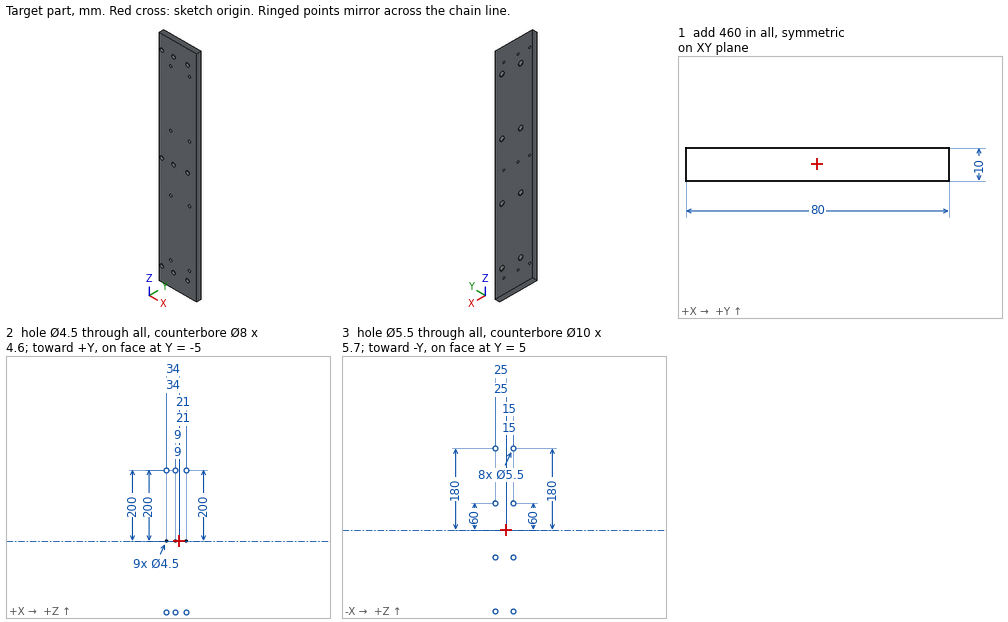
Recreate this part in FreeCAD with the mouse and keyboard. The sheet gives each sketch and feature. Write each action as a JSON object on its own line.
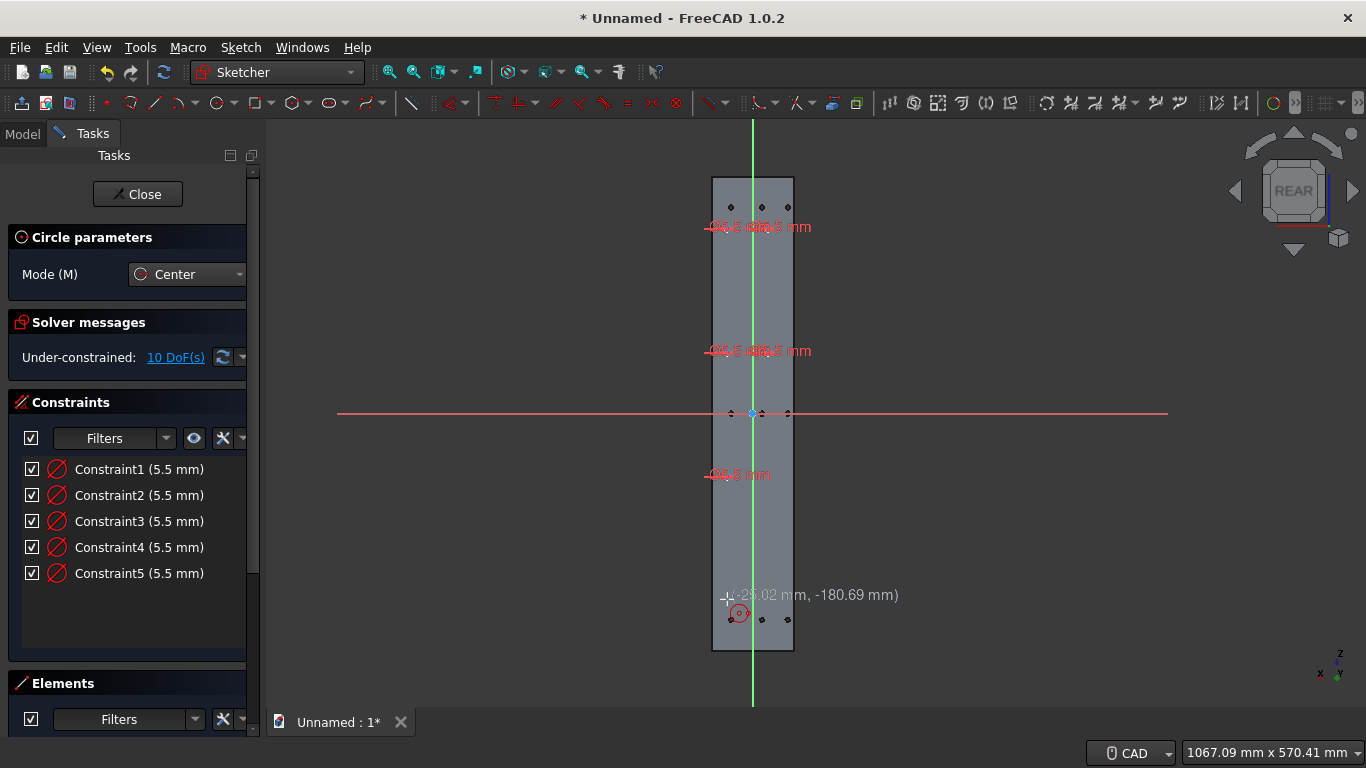
{"action": "left_click", "coordinate": [727, 599]}
{"action": "mouse_move", "coordinate": [729, 597]}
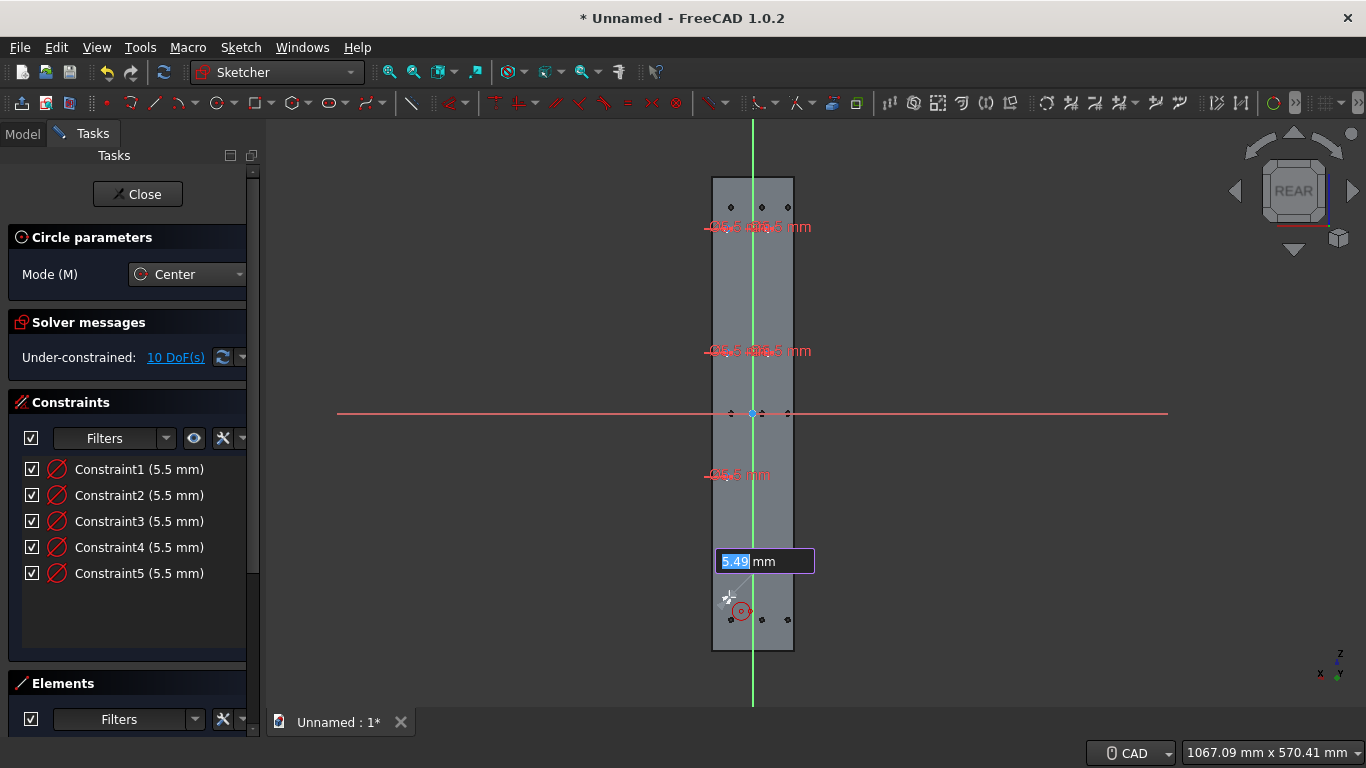
{"action": "type", "text": "5.5"}
{"action": "key", "text": "Return"}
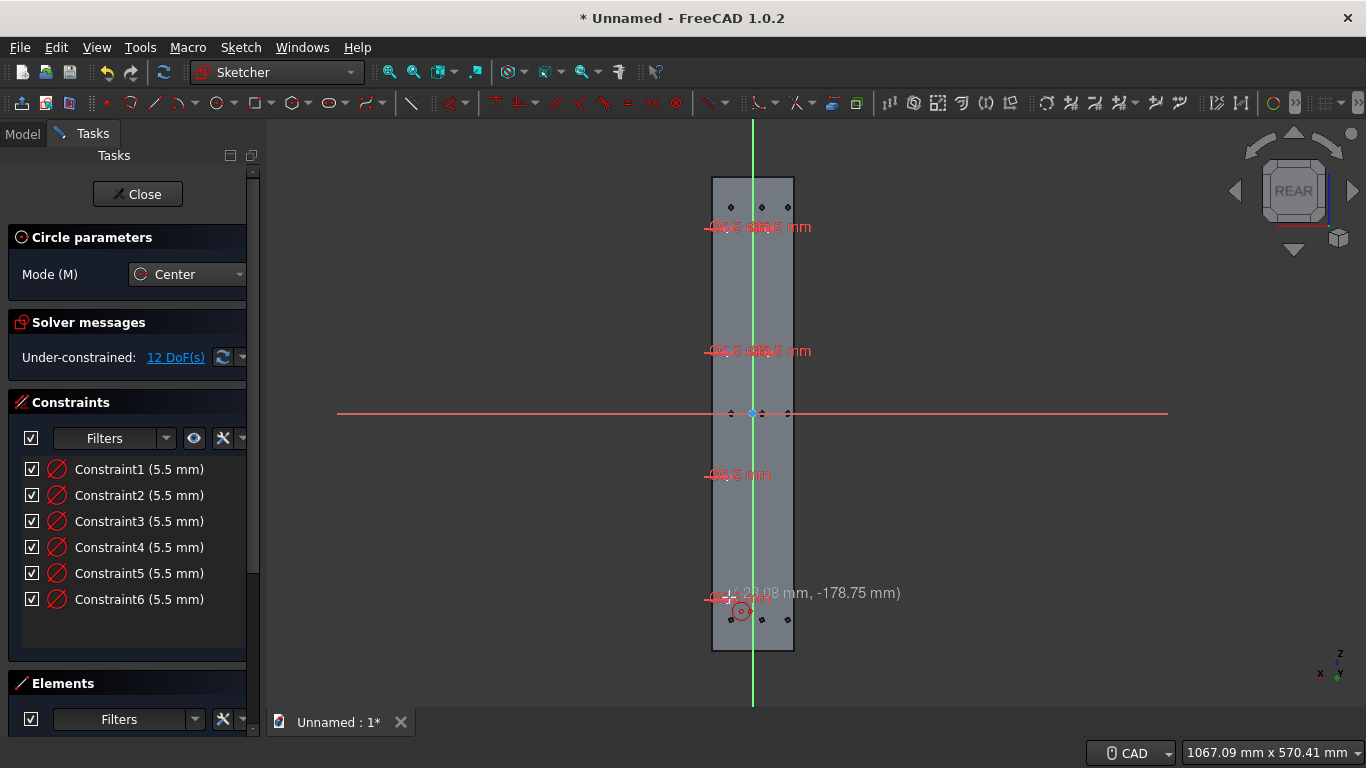
{"action": "scroll", "coordinate": [768, 599], "scroll_direction": "up", "scroll_amount": 11}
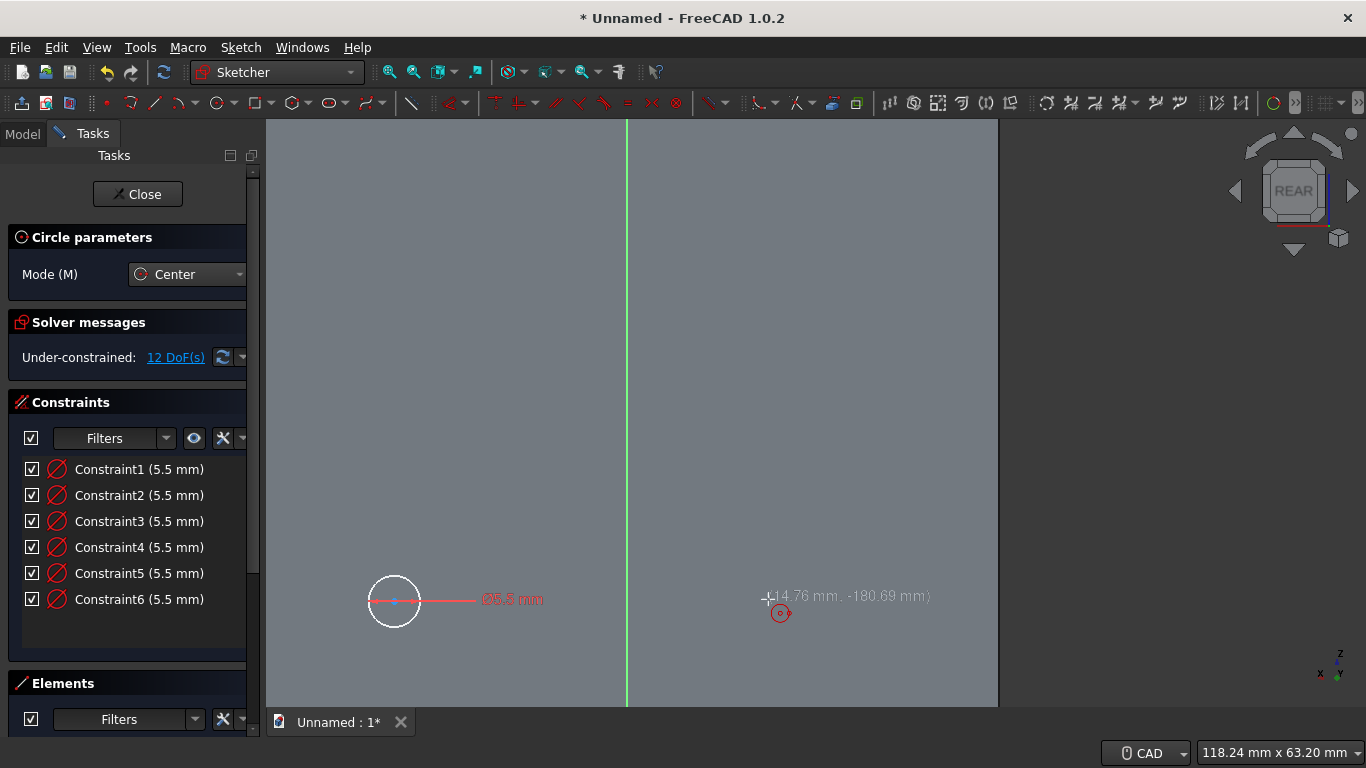
{"action": "scroll", "coordinate": [768, 599], "scroll_direction": "down", "scroll_amount": 11}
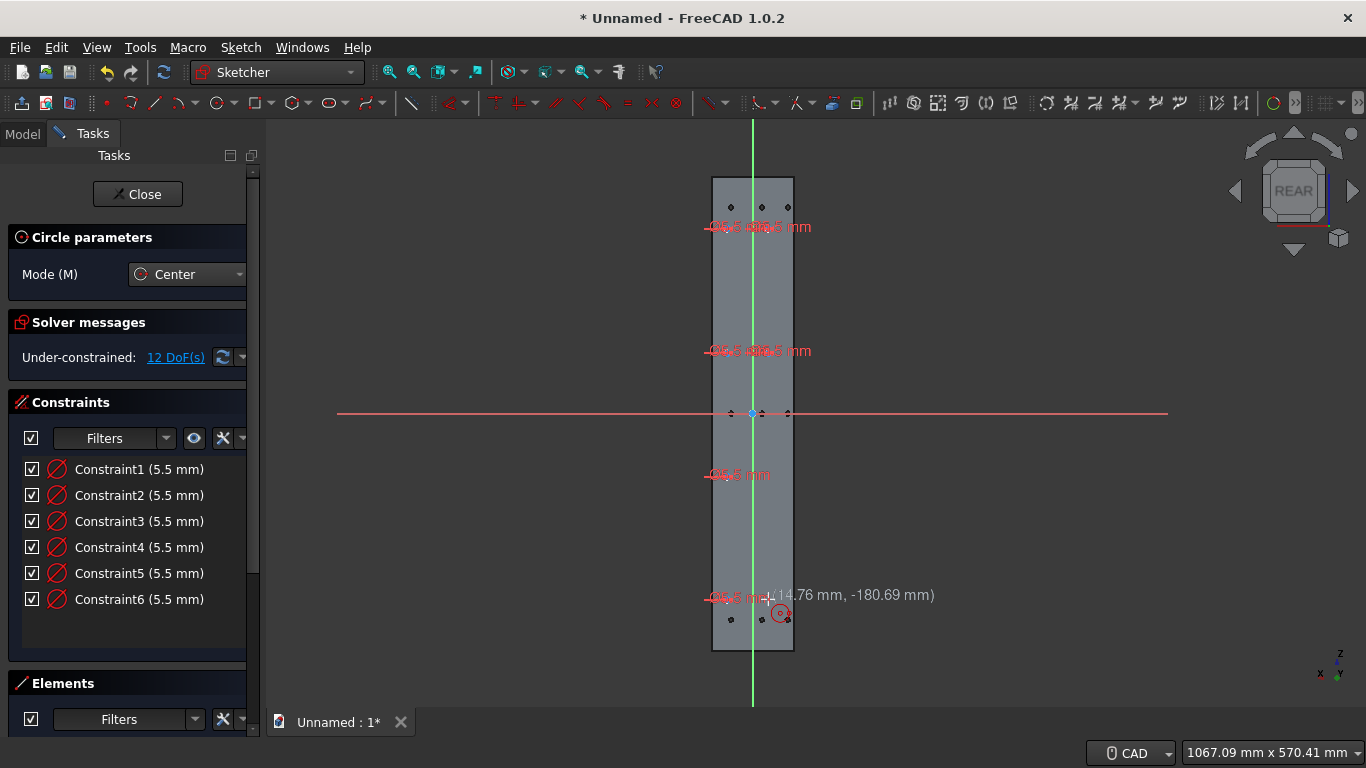
{"action": "left_click", "coordinate": [768, 599]}
{"action": "mouse_move", "coordinate": [770, 597]}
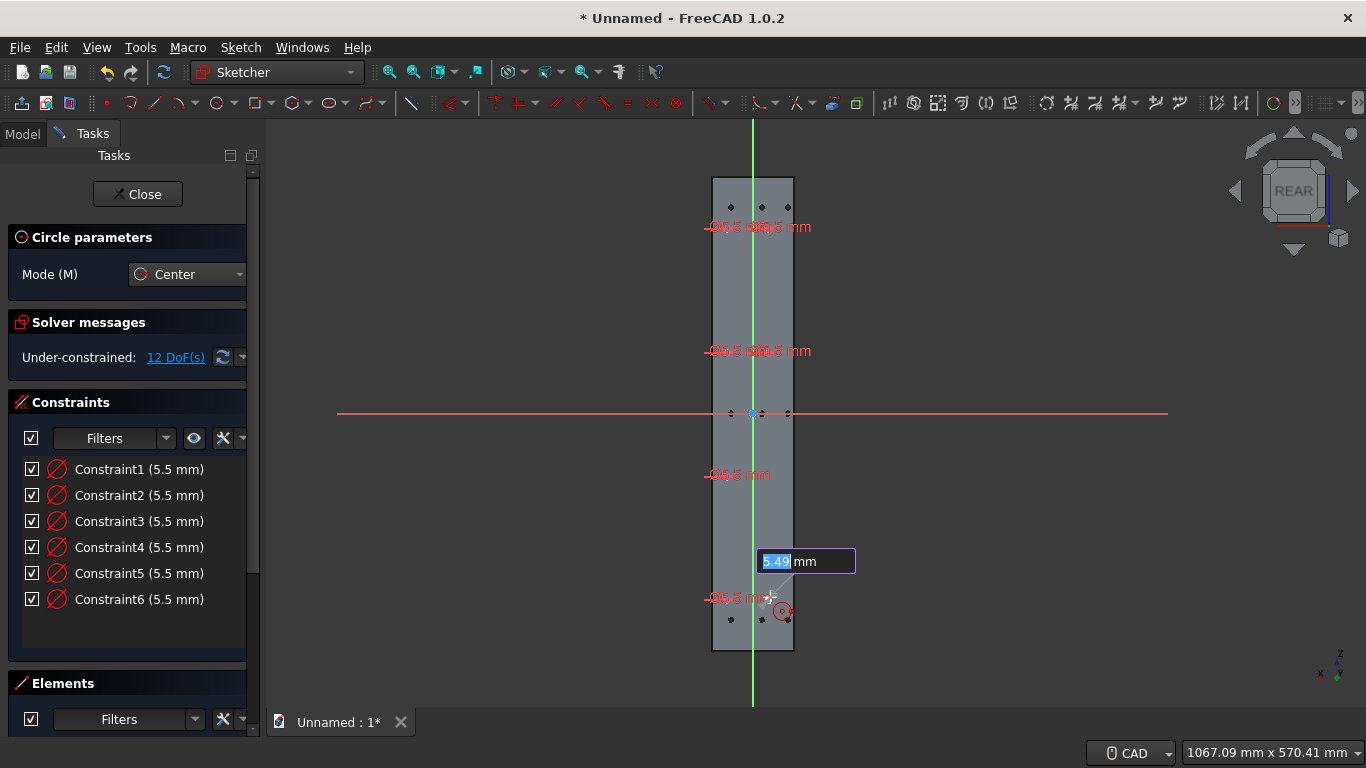
{"action": "type", "text": "5.5"}
{"action": "key", "text": "Return"}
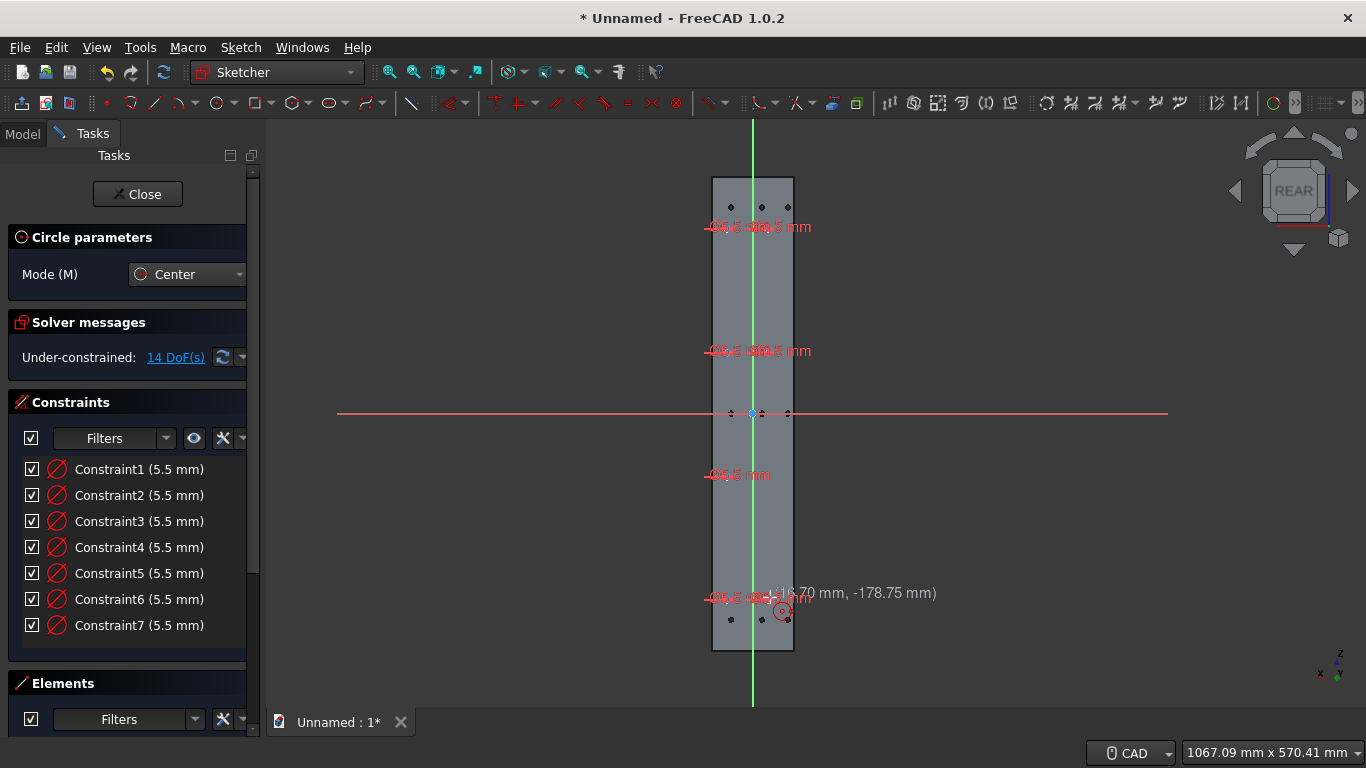
{"action": "scroll", "coordinate": [768, 476], "scroll_direction": "up", "scroll_amount": 11}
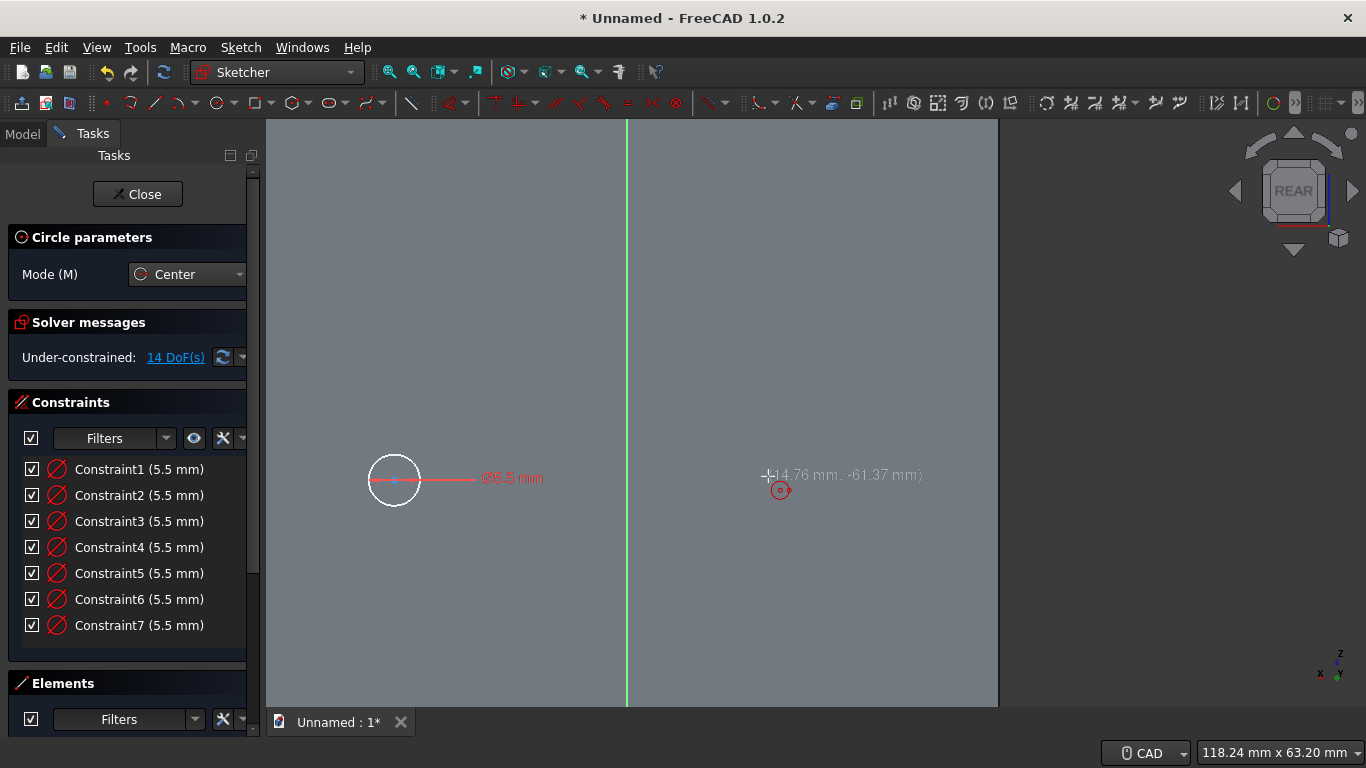
{"action": "scroll", "coordinate": [768, 476], "scroll_direction": "down", "scroll_amount": 11}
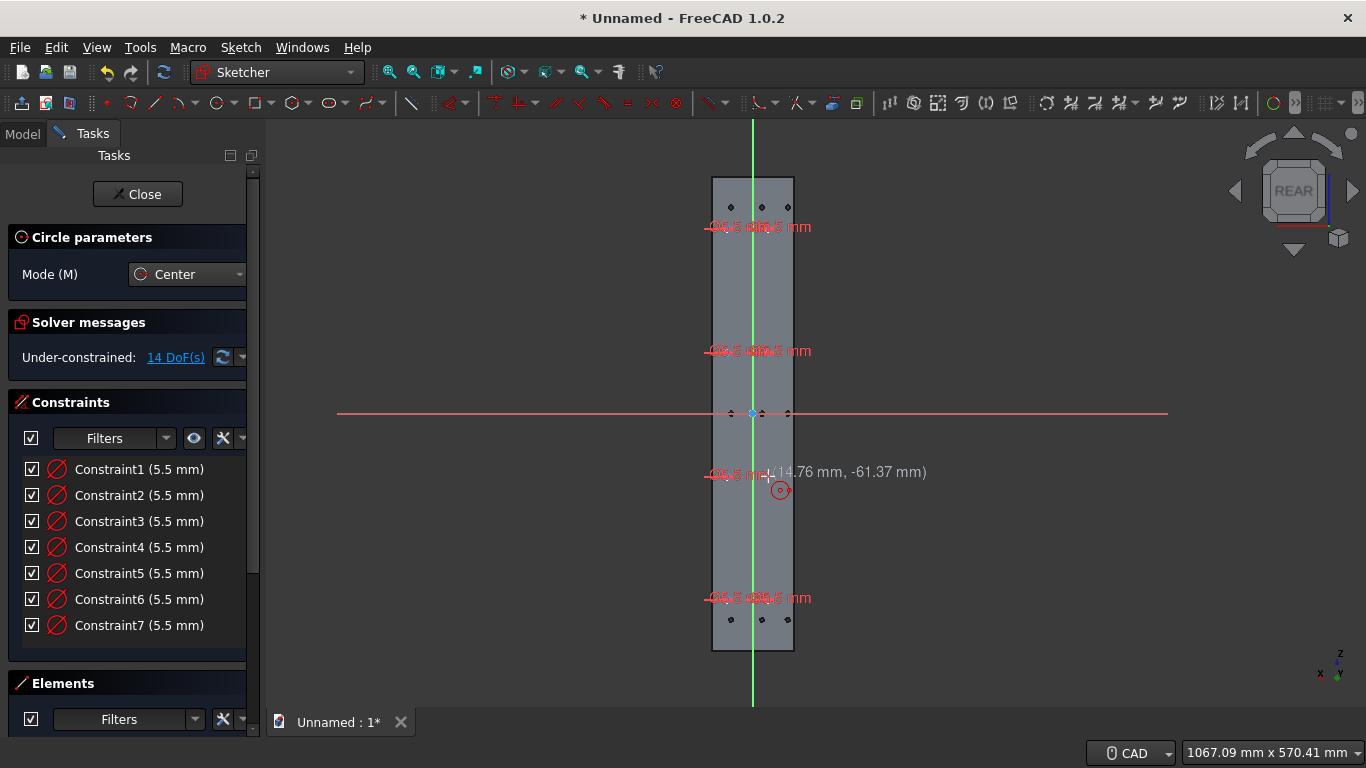
{"action": "left_click", "coordinate": [768, 476]}
{"action": "mouse_move", "coordinate": [770, 474]}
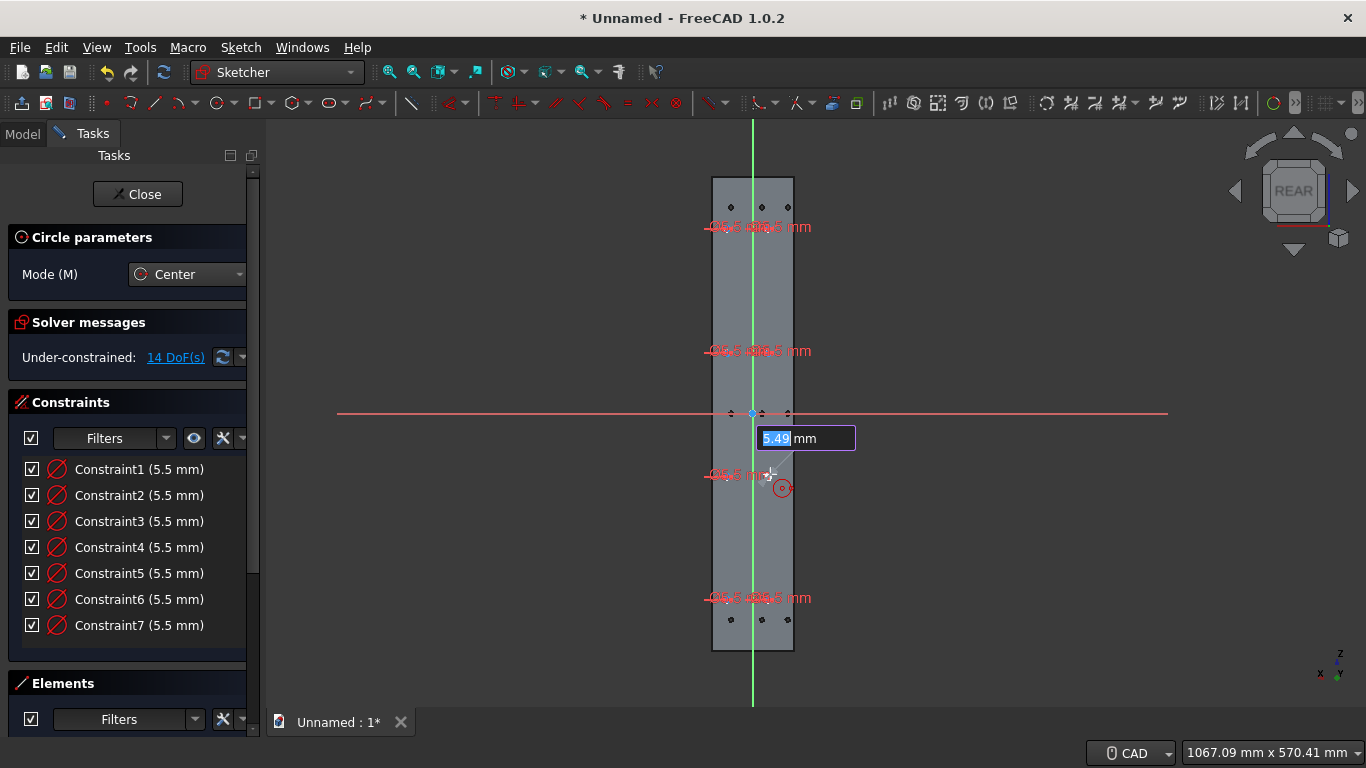
{"action": "type", "text": "5.5"}
{"action": "key", "text": "Return"}
{"action": "key", "text": "Escape"}